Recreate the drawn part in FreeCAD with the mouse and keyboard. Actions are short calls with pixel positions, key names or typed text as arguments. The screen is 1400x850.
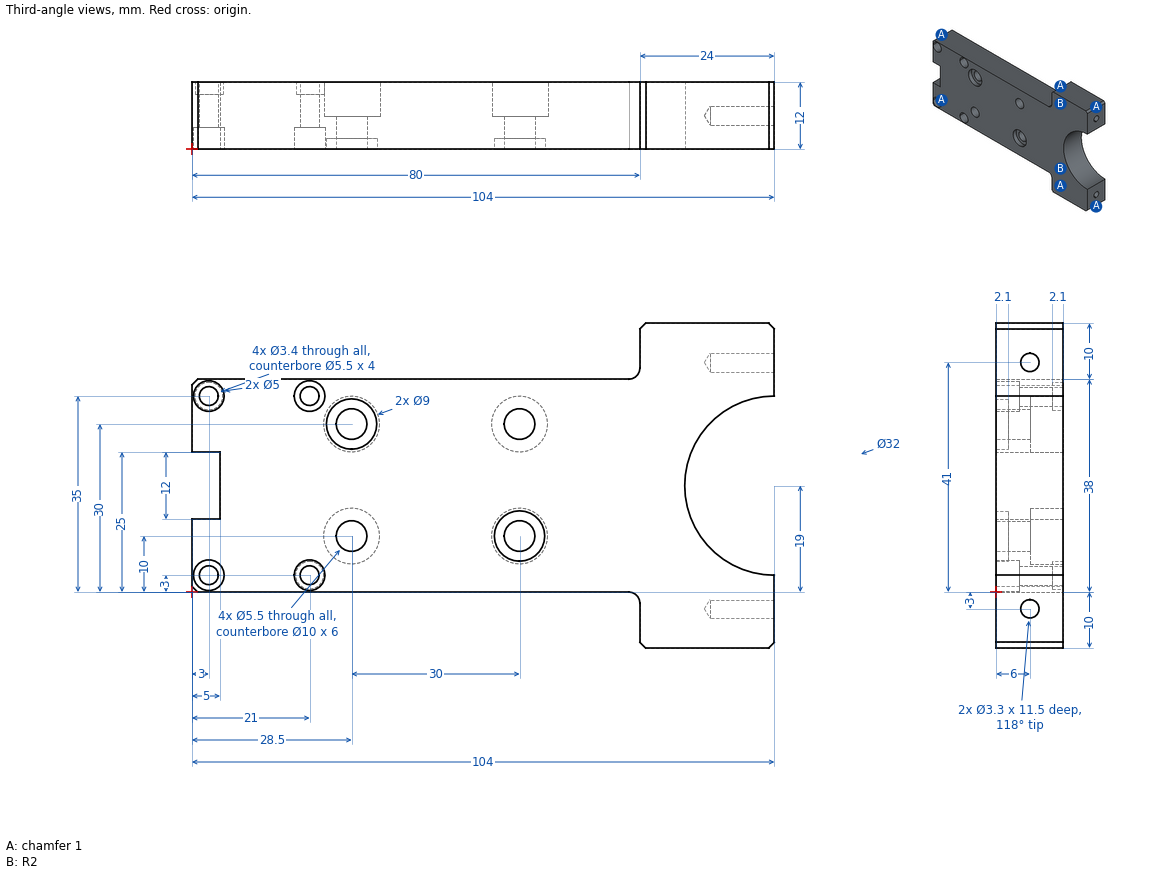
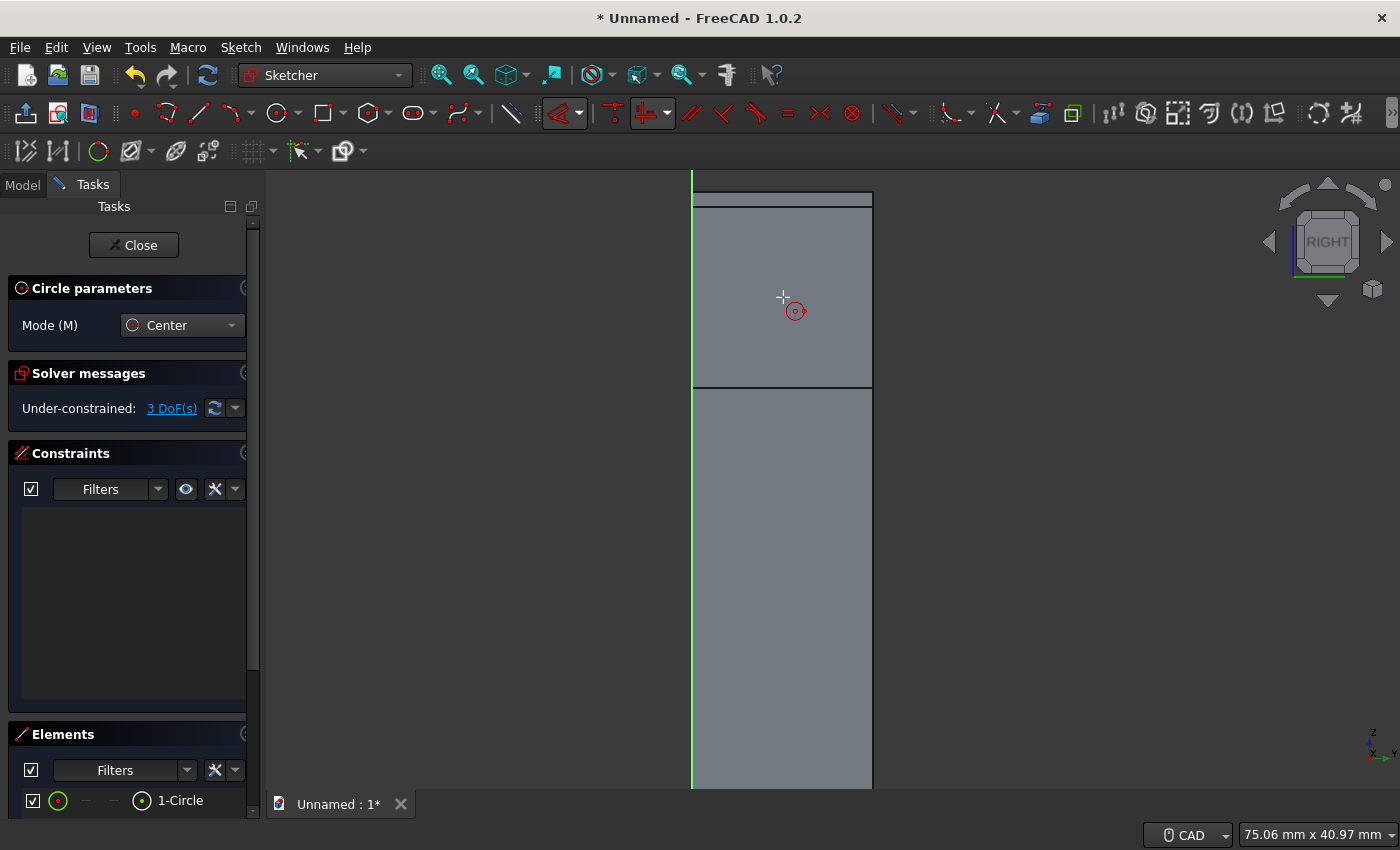
click(782, 297)
click(800, 280)
key(Escape)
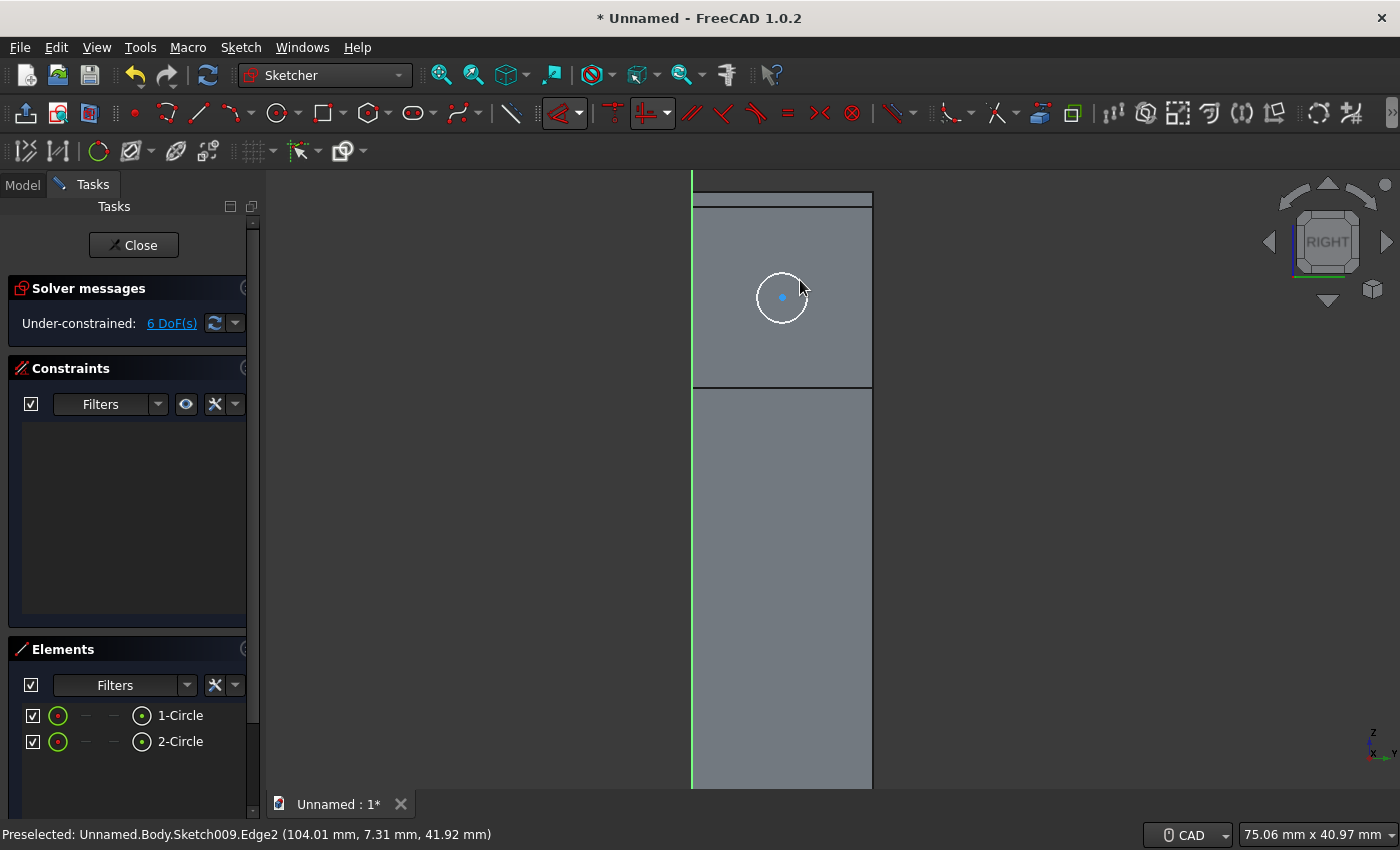
scroll(783, 297, down, 3)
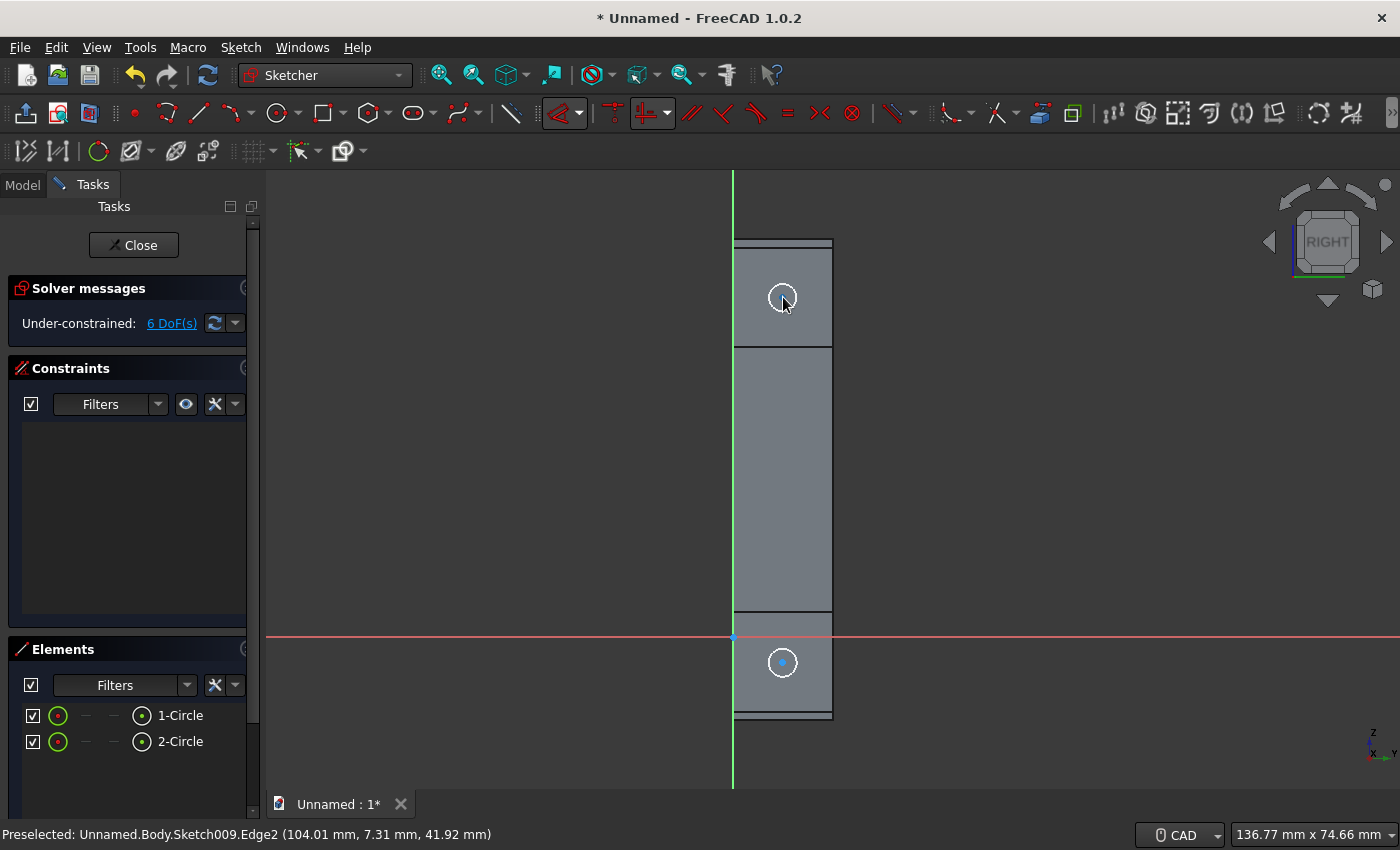
click(793, 653)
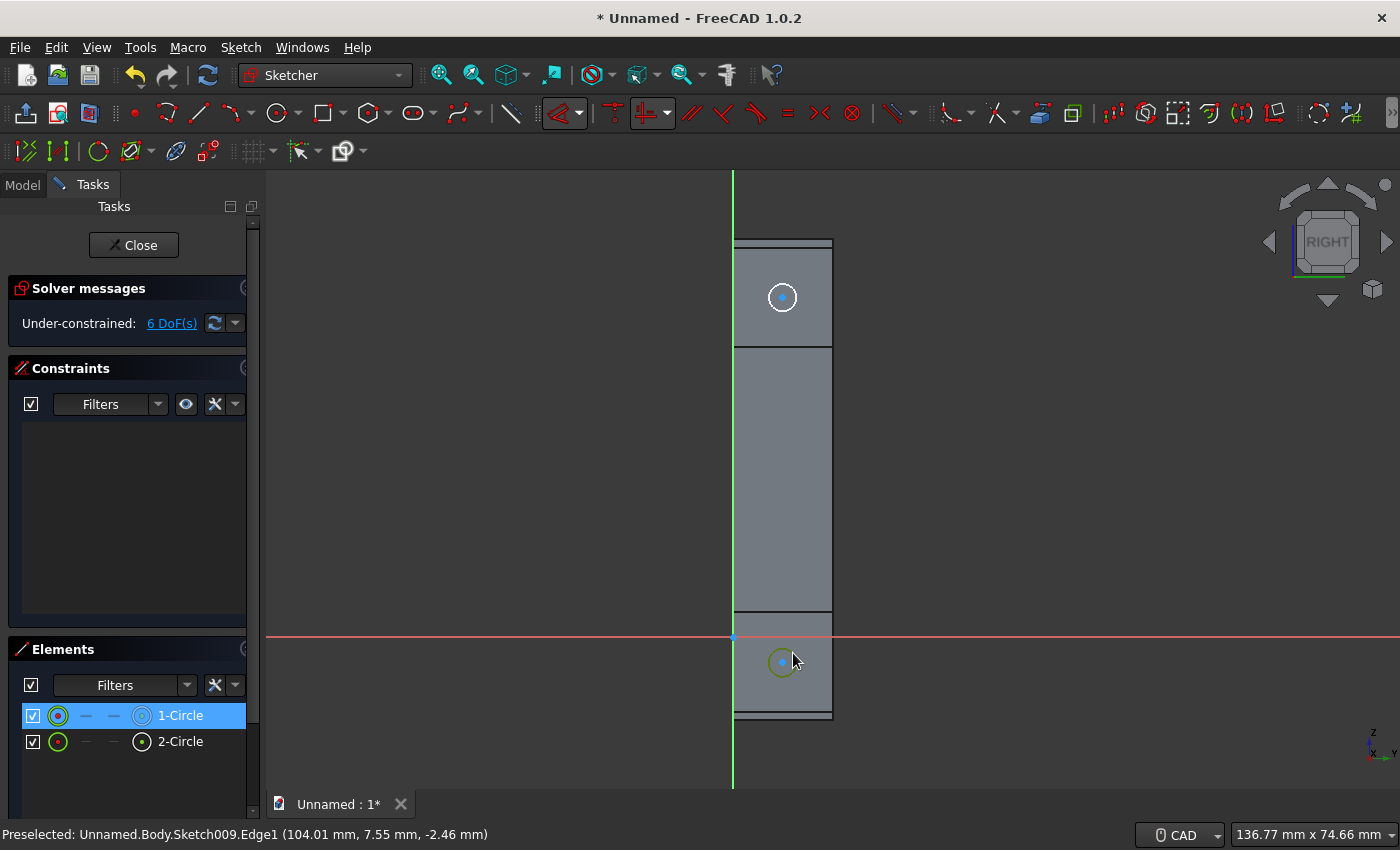
click(792, 288)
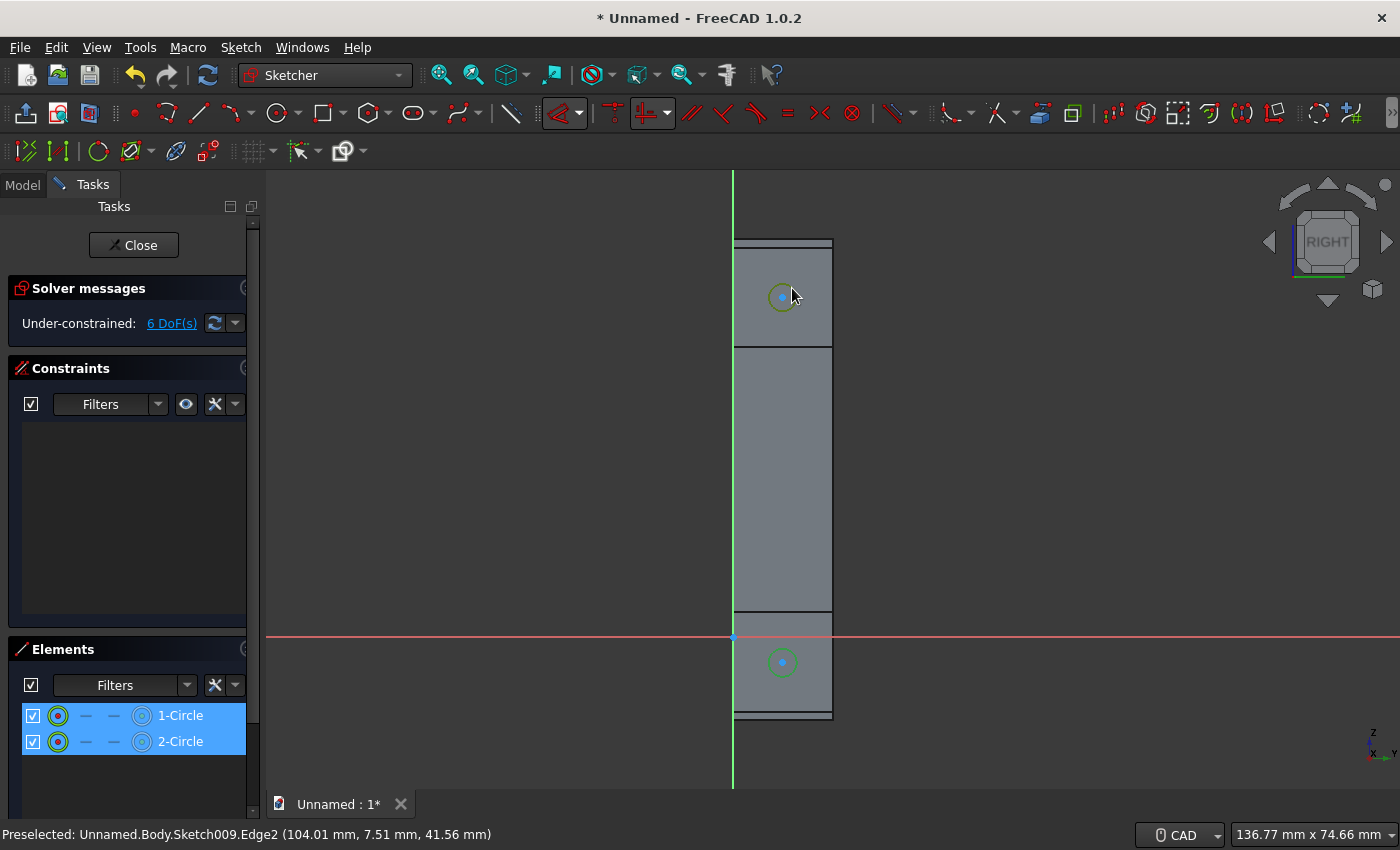
click(788, 114)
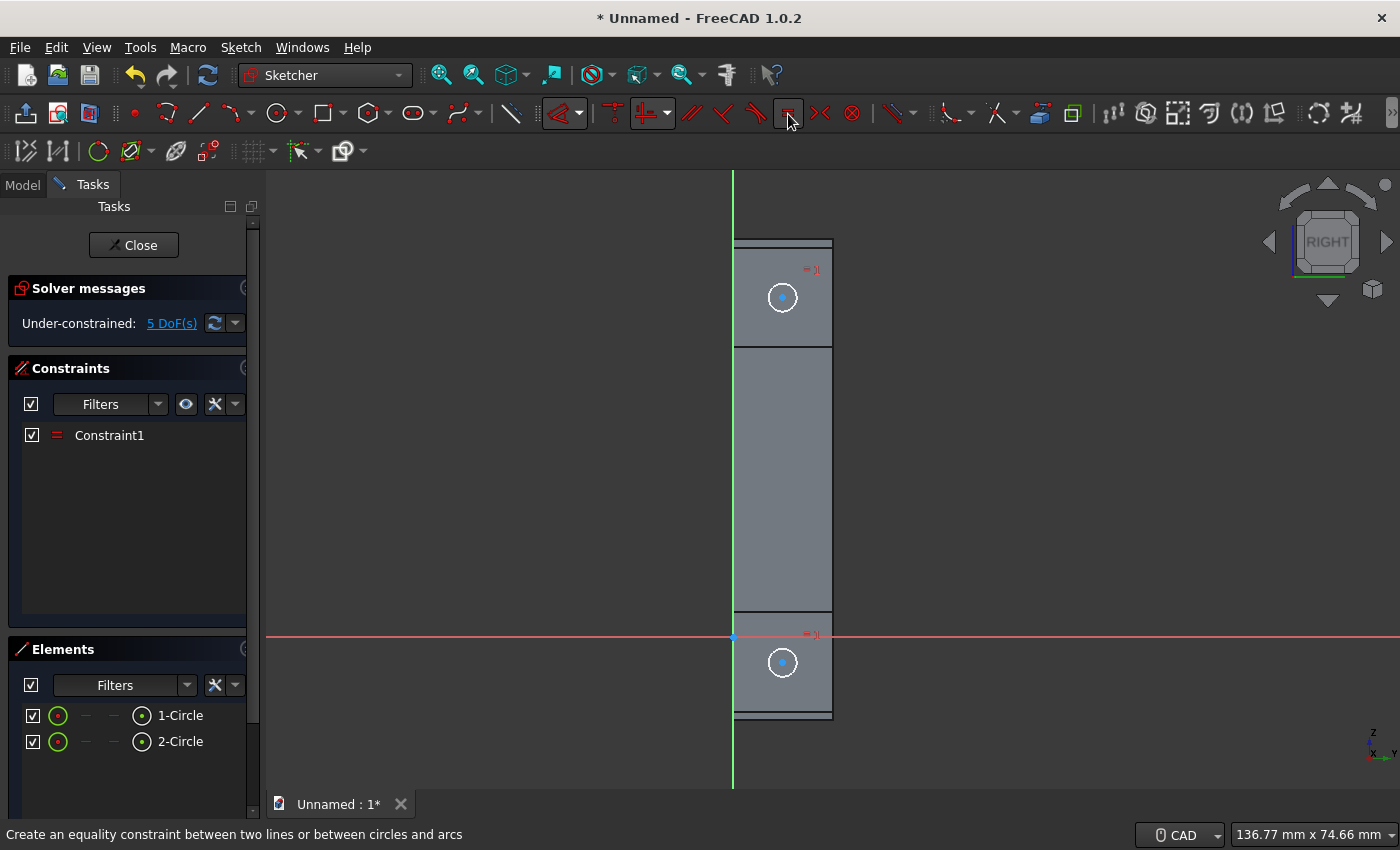
click(783, 663)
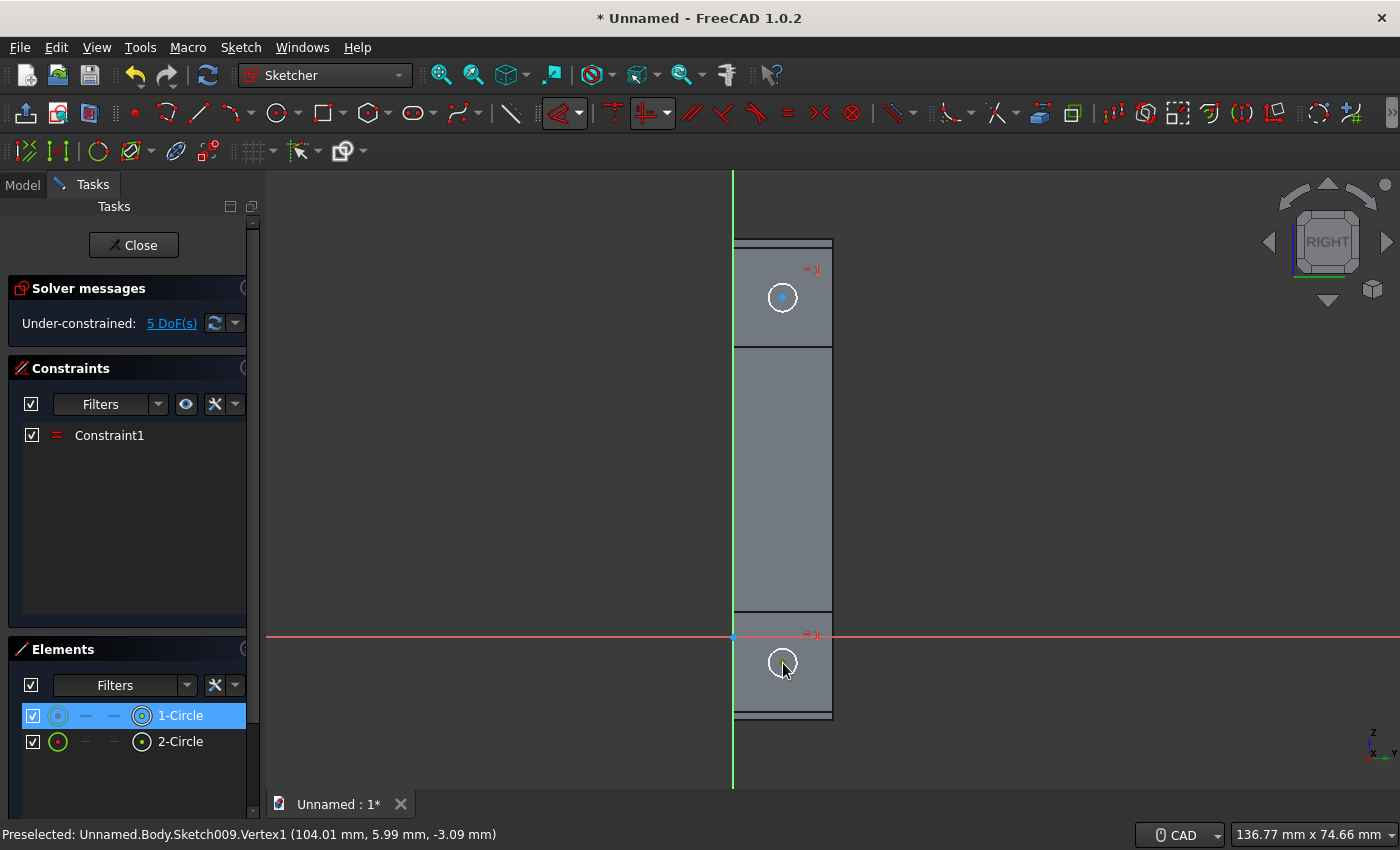
click(783, 298)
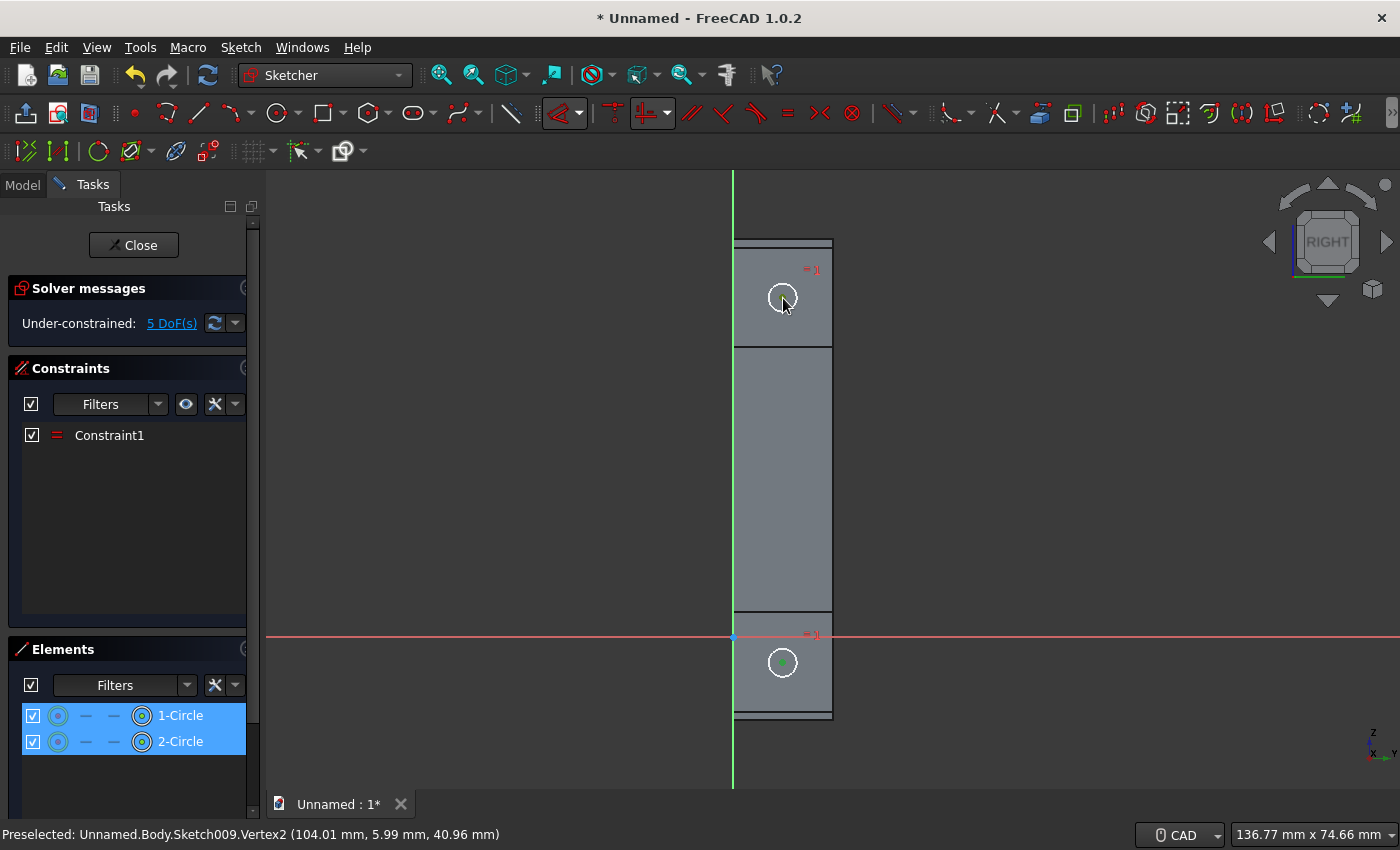
click(670, 114)